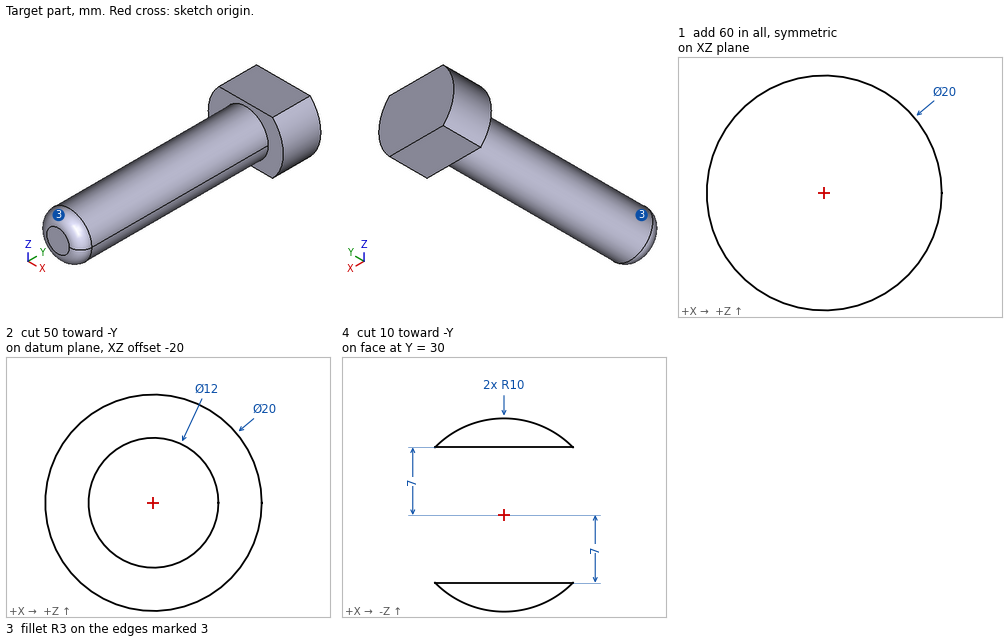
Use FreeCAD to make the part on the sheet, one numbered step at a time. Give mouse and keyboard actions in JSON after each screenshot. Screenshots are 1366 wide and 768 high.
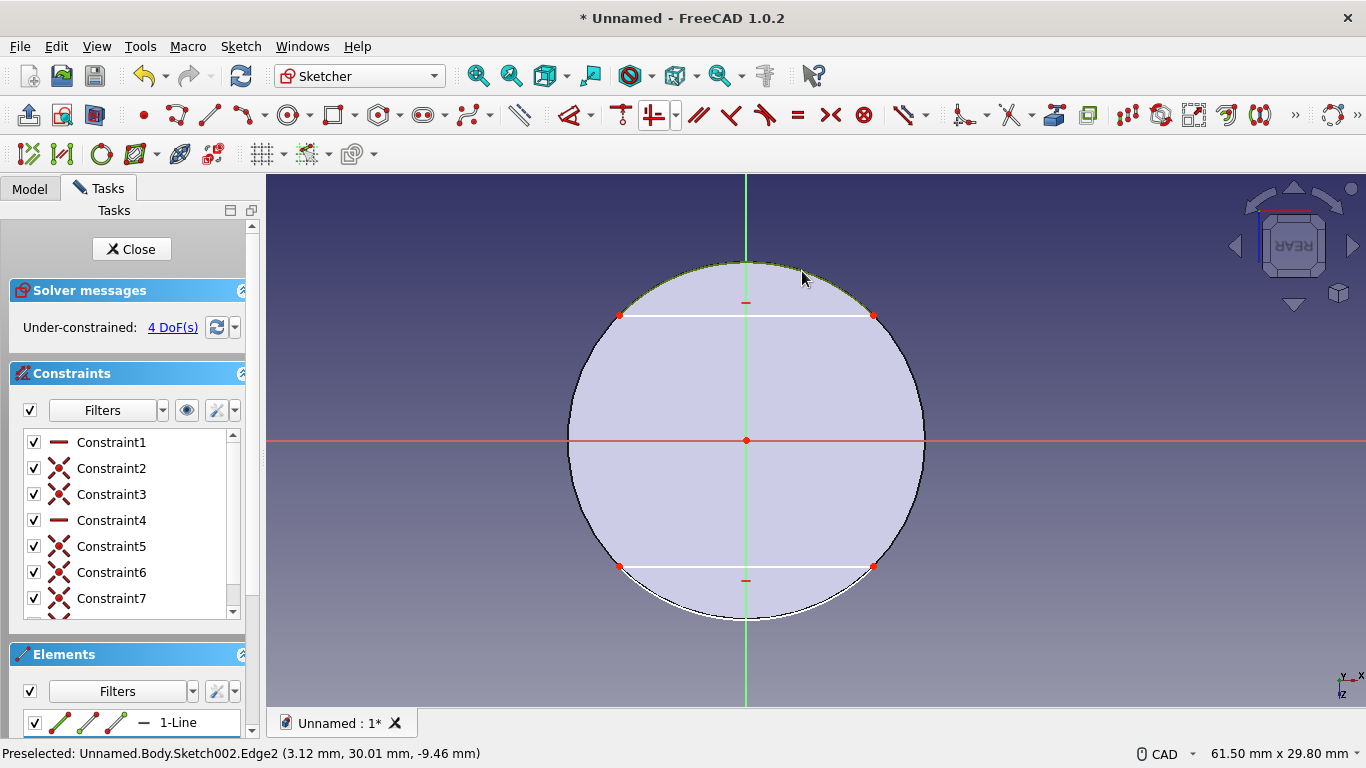
{"action": "left_click", "coordinate": [691, 611]}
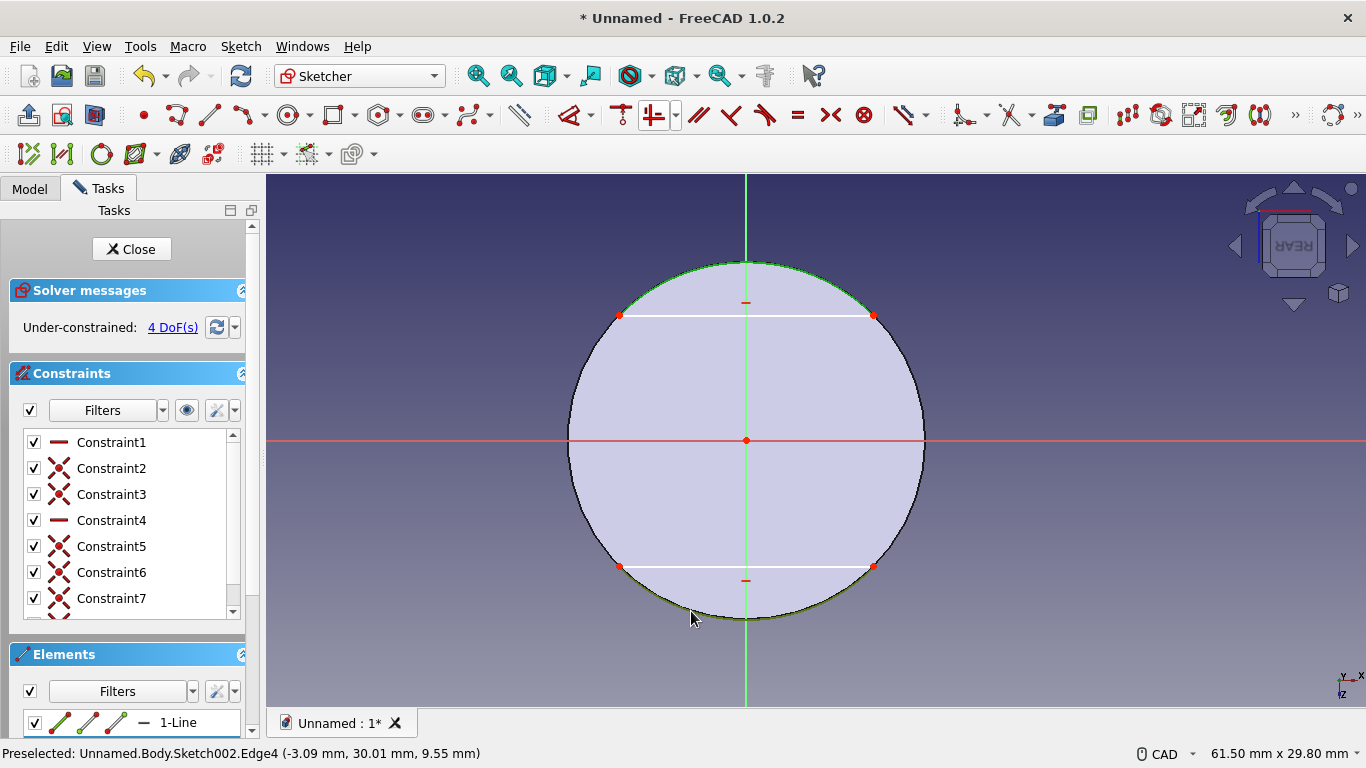
{"action": "key", "text": "e"}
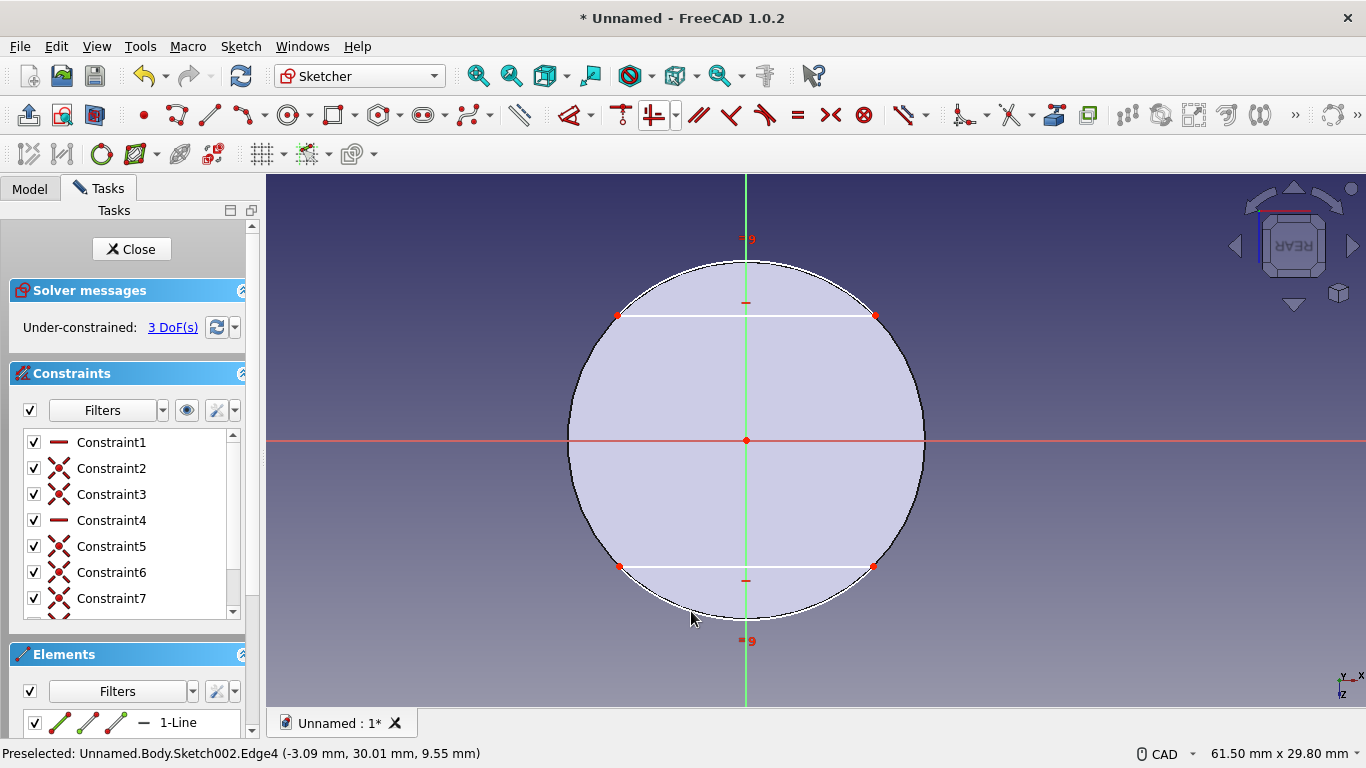
{"action": "left_click", "coordinate": [568, 116]}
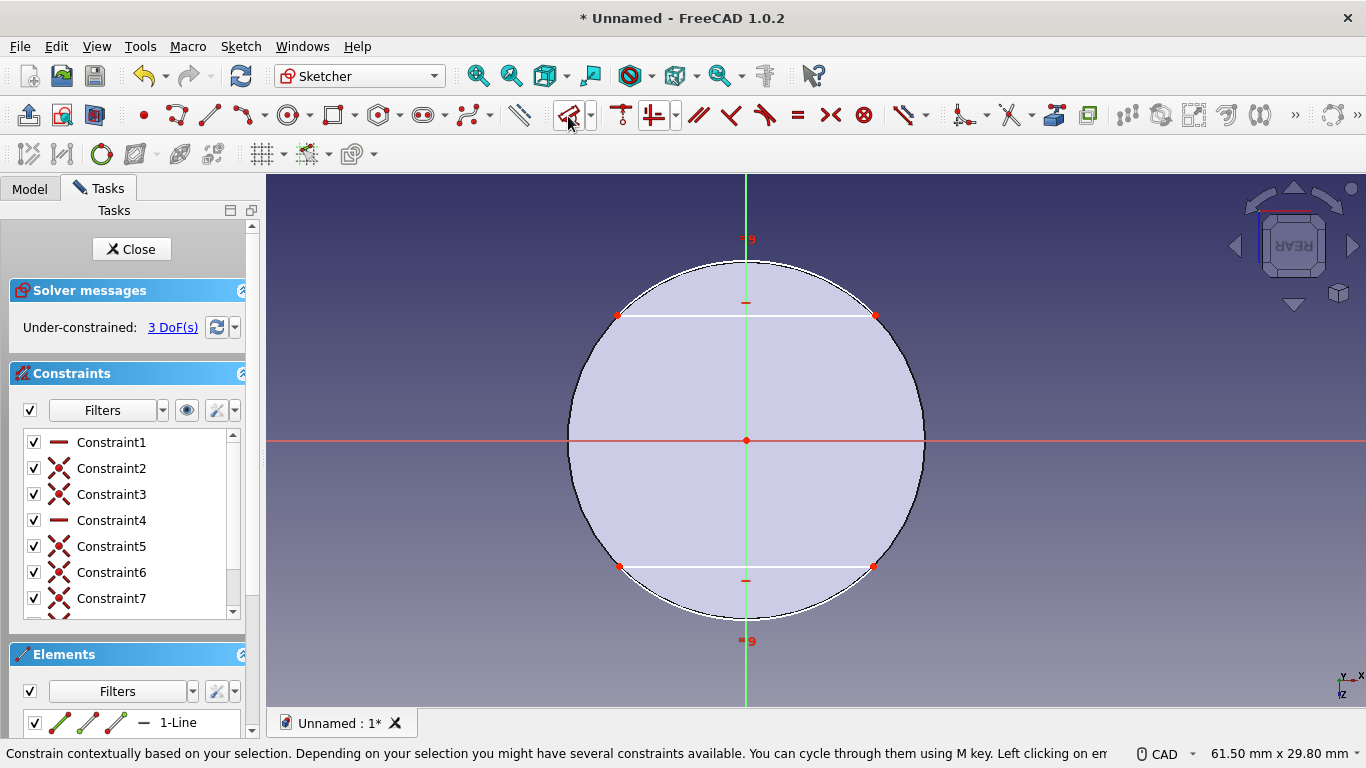
{"action": "left_click", "coordinate": [803, 270]}
{"action": "left_click", "coordinate": [813, 240]}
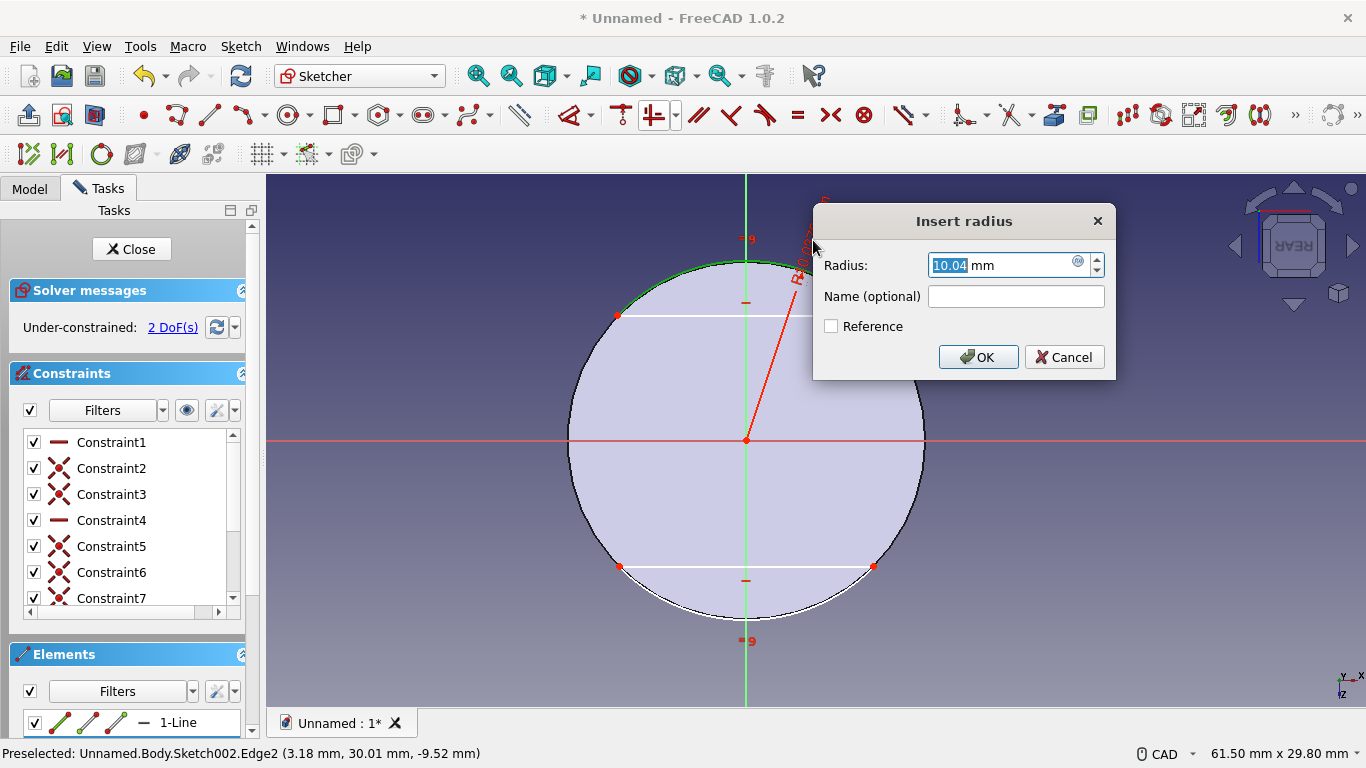
{"action": "type", "text": "10"}
{"action": "key", "text": "Return"}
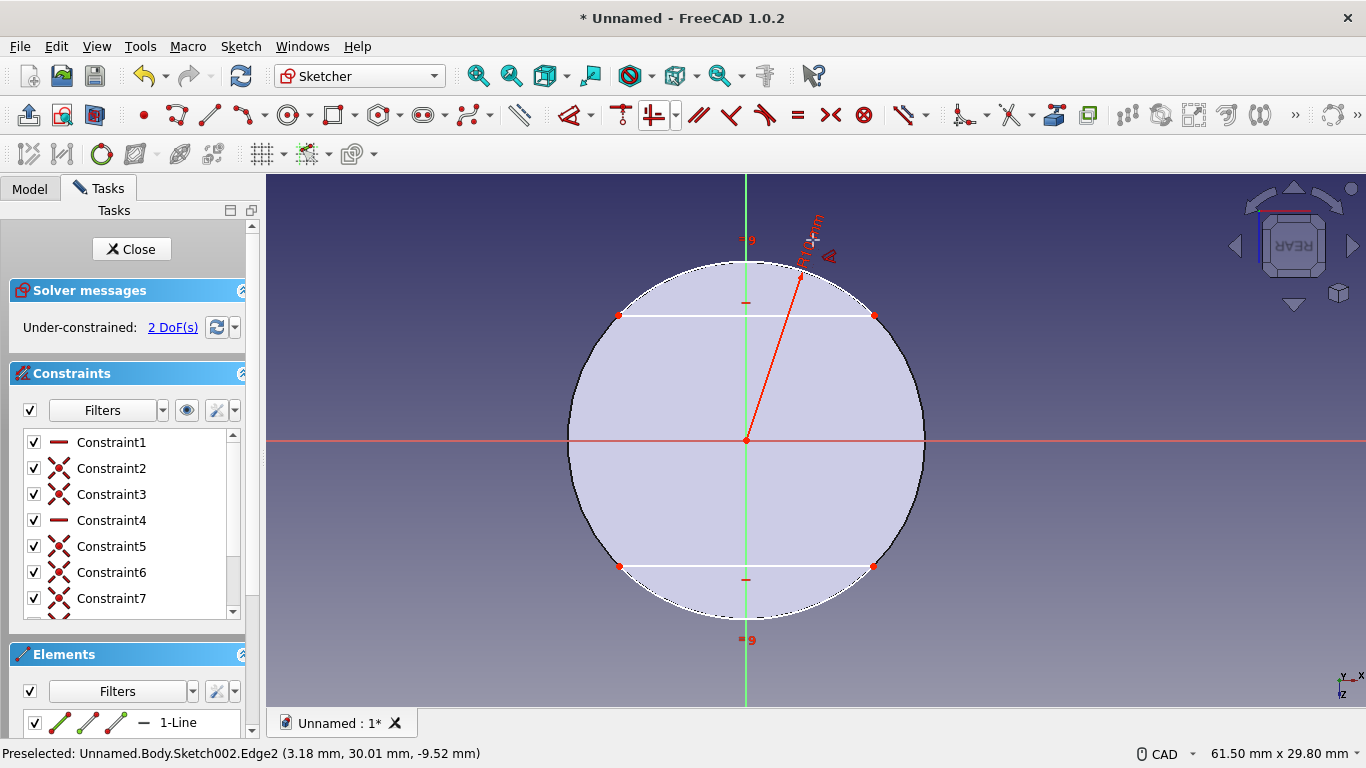
{"action": "left_click", "coordinate": [618, 316]}
{"action": "left_click", "coordinate": [584, 378]}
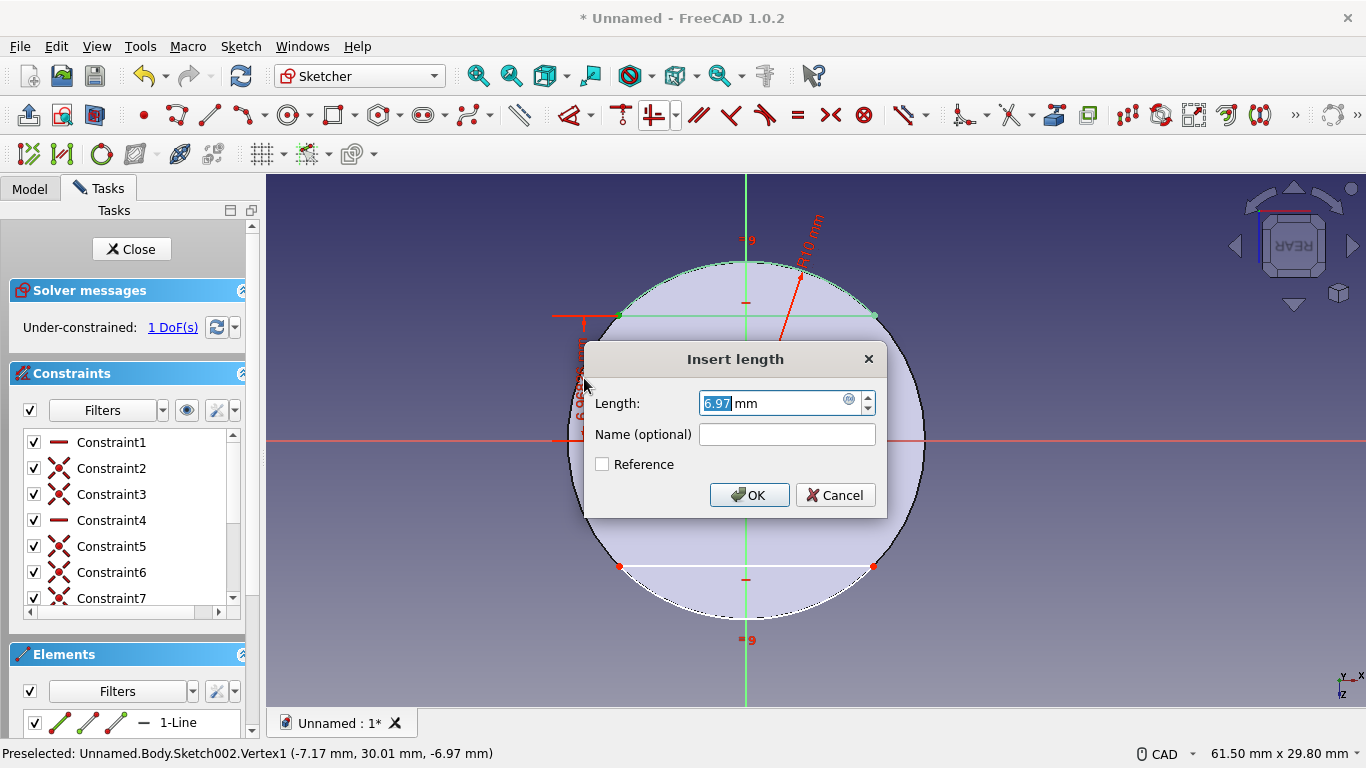
{"action": "type", "text": "7"}
{"action": "key", "text": "Return"}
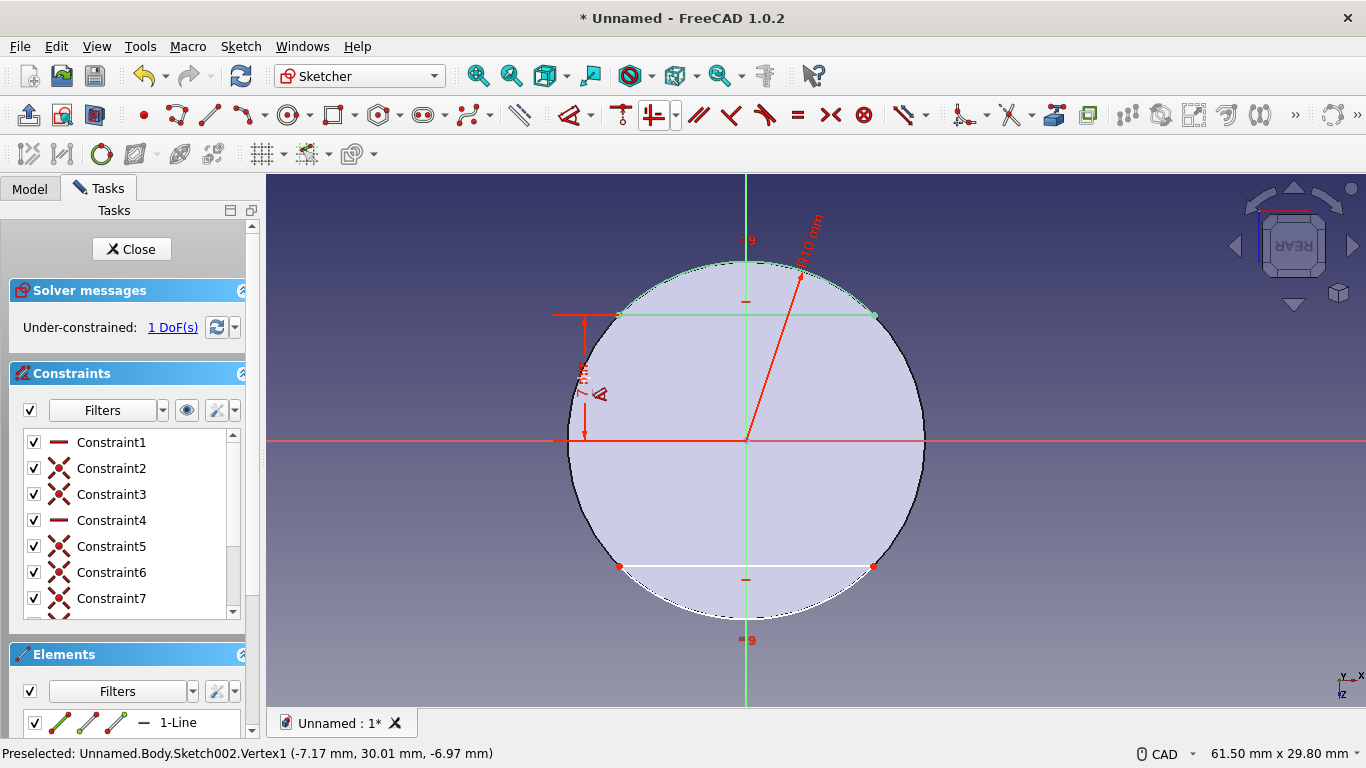
{"action": "left_click", "coordinate": [874, 566]}
{"action": "left_click", "coordinate": [908, 503]}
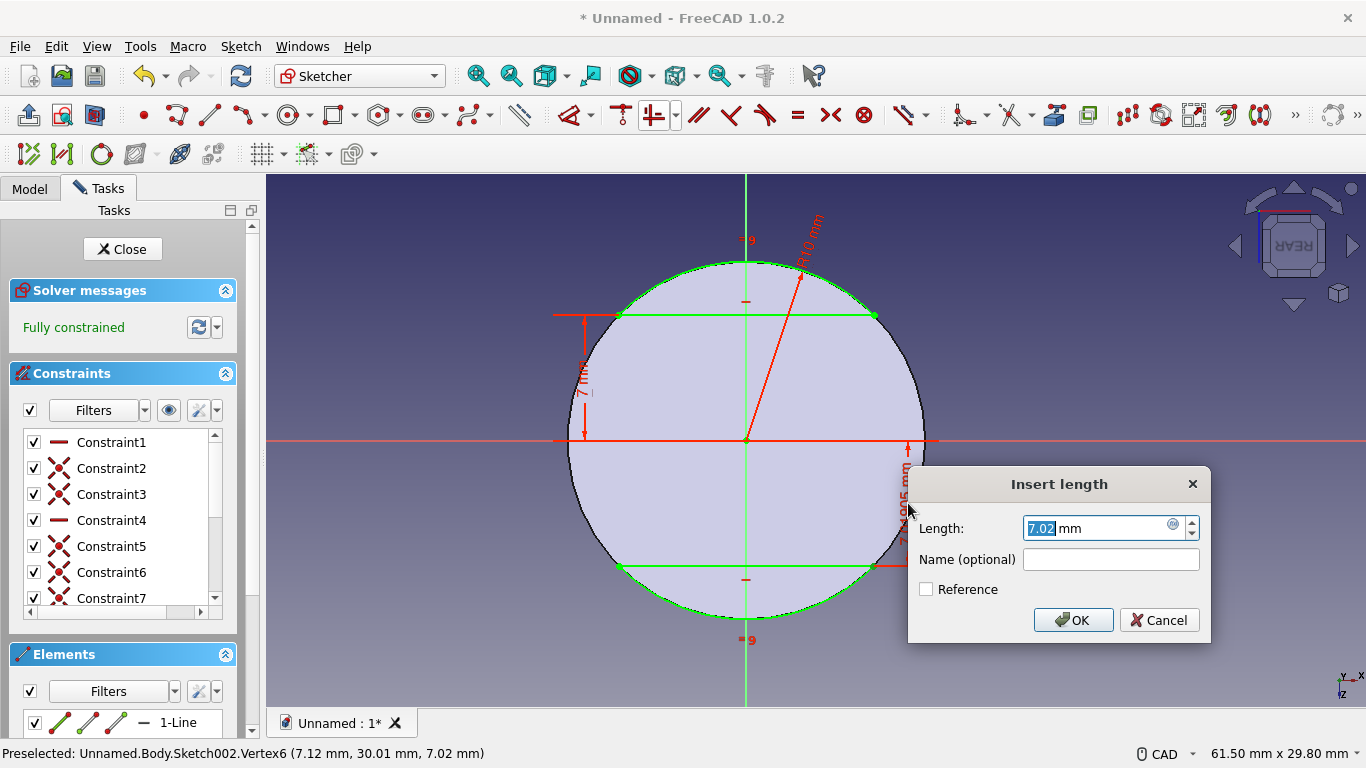
{"action": "type", "text": "7"}
{"action": "key", "text": "Return"}
{"action": "key", "text": "Escape"}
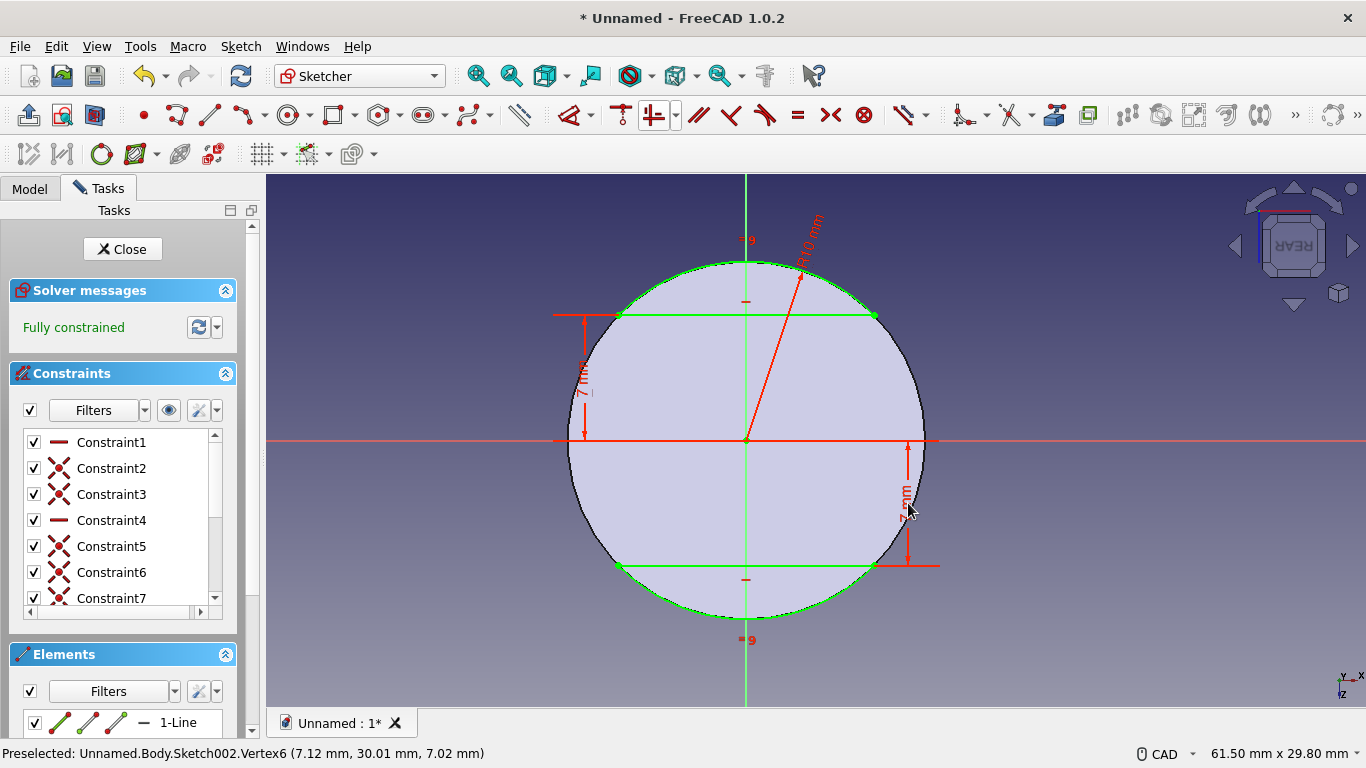
{"action": "left_click", "coordinate": [123, 249]}